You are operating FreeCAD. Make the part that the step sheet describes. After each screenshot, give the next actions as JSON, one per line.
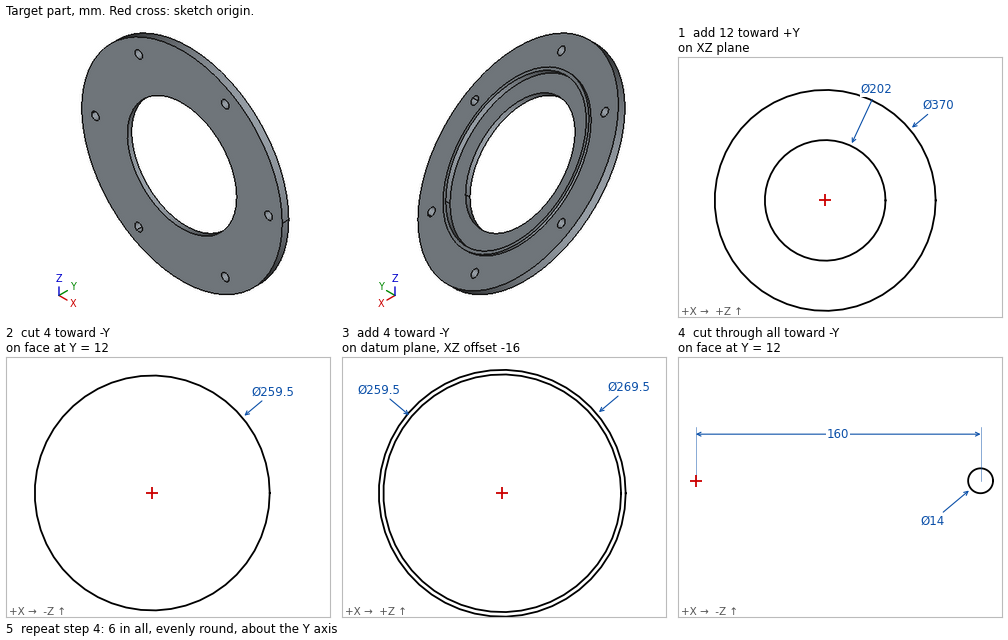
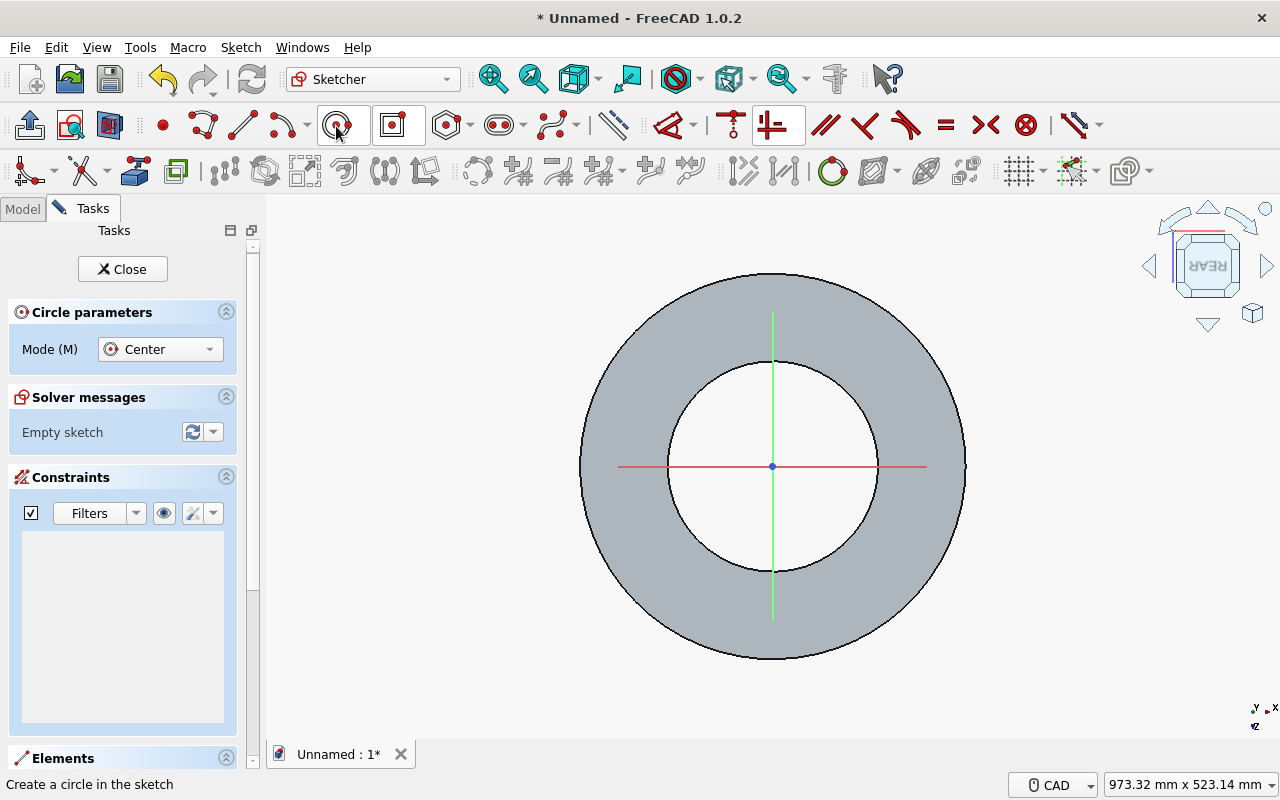
{"action": "left_click", "coordinate": [773, 466]}
{"action": "mouse_move", "coordinate": [868, 371]}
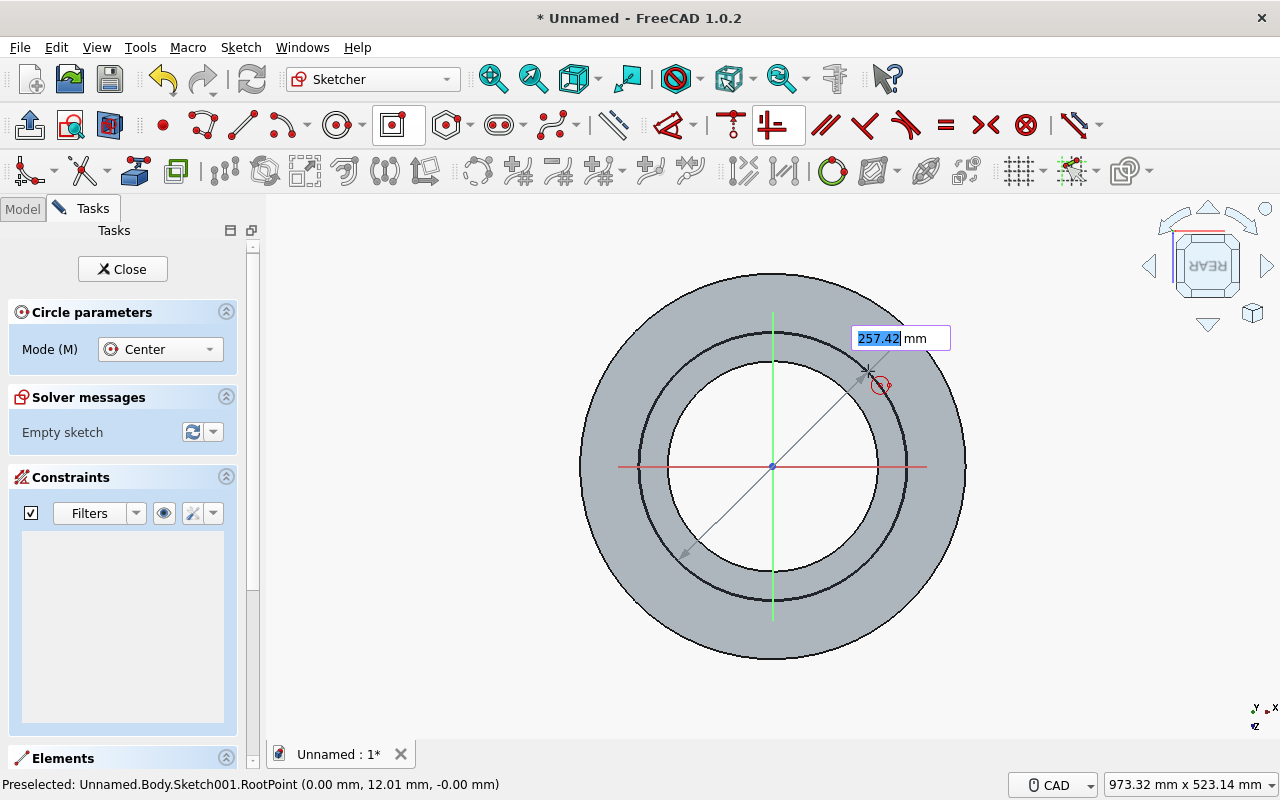
{"action": "type", "text": "259.5"}
{"action": "key", "text": "Return"}
{"action": "key", "text": "Escape"}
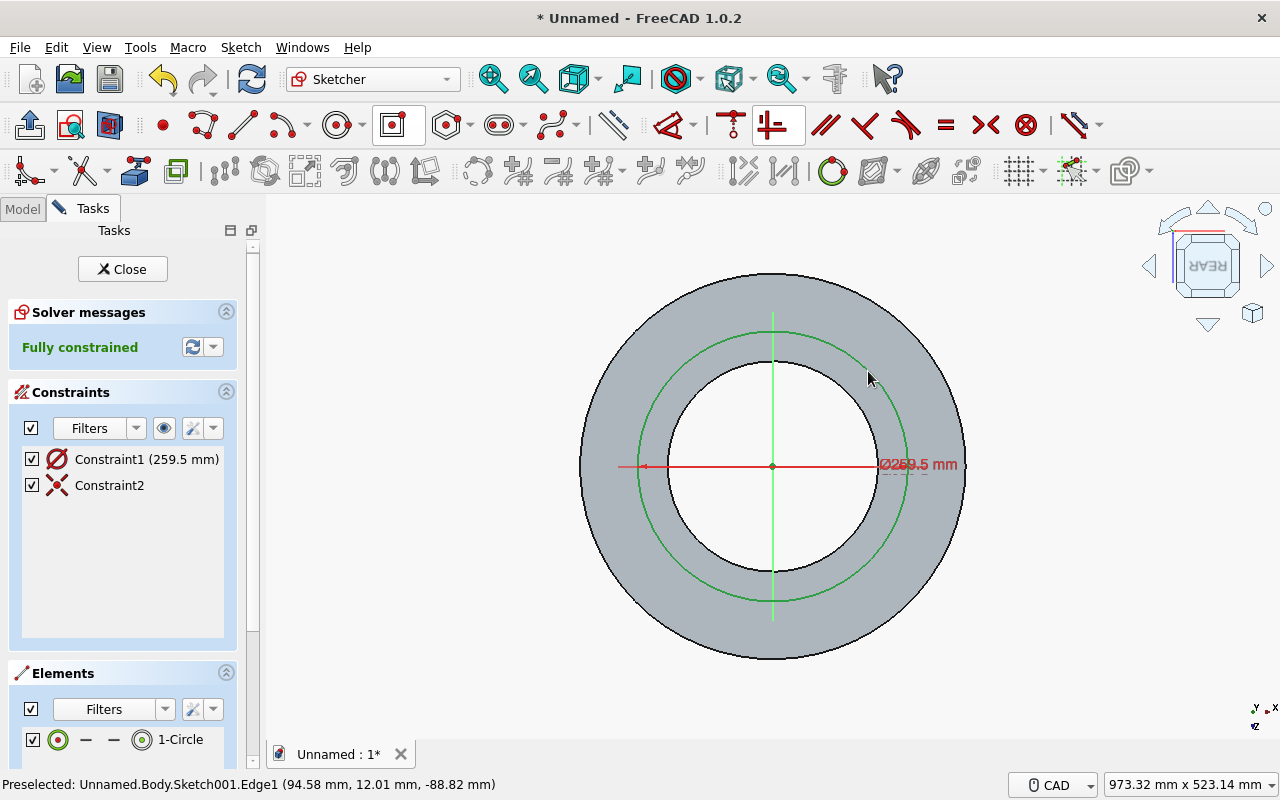
{"action": "left_click", "coordinate": [123, 269]}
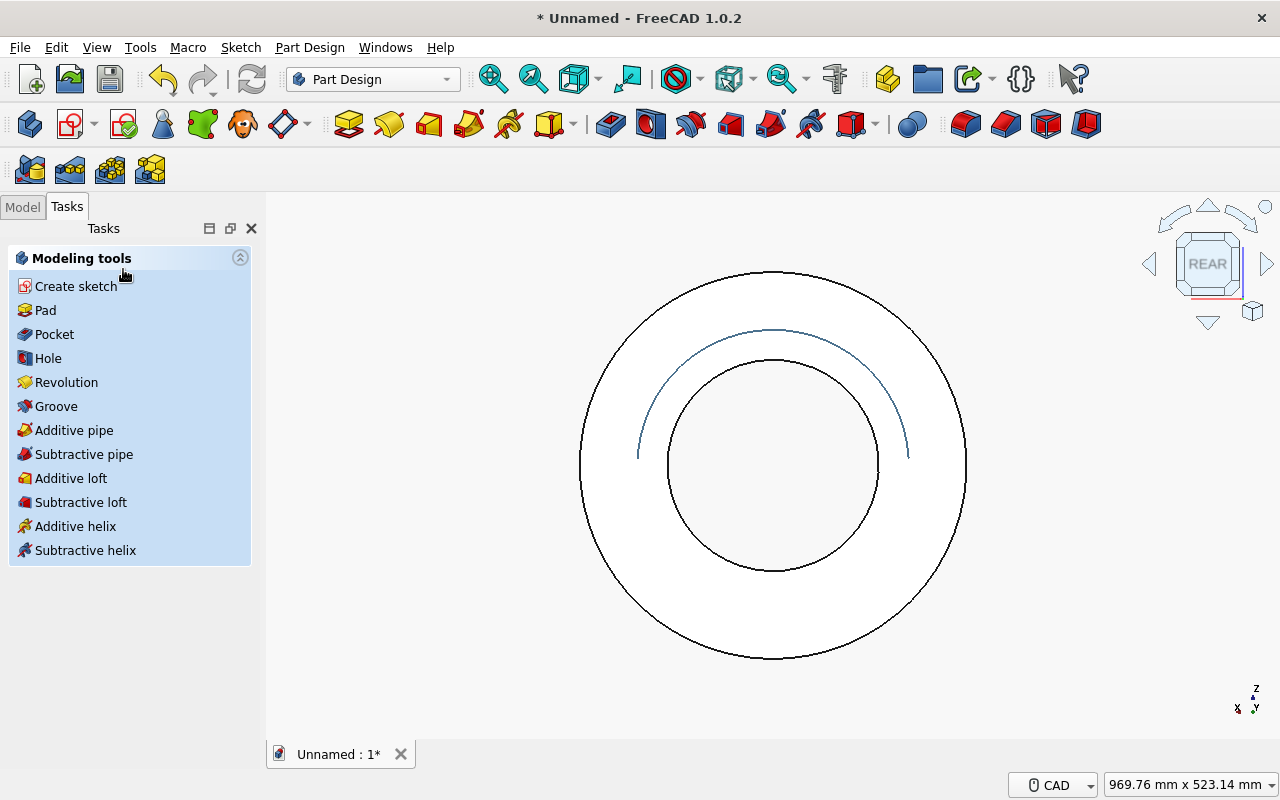
{"action": "left_click", "coordinate": [612, 124]}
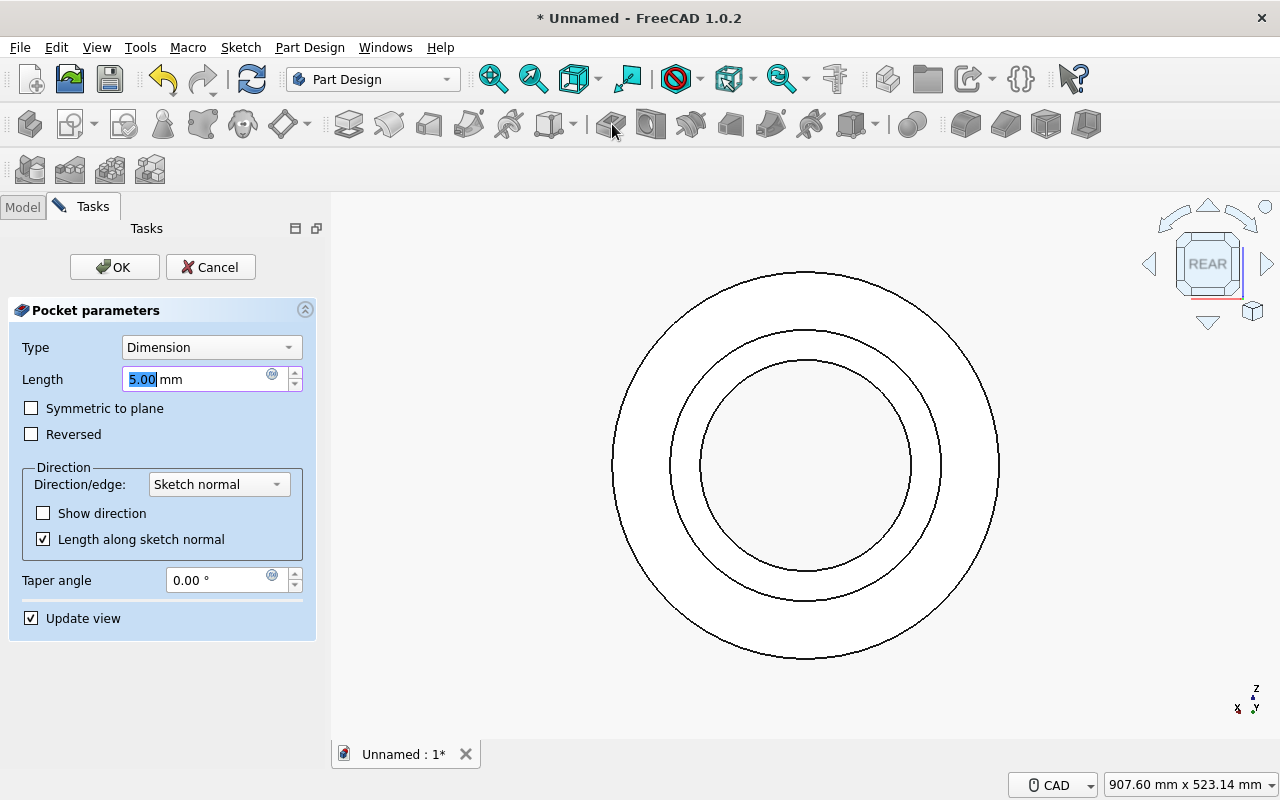
{"action": "type", "text": "4"}
{"action": "key", "text": "Tab"}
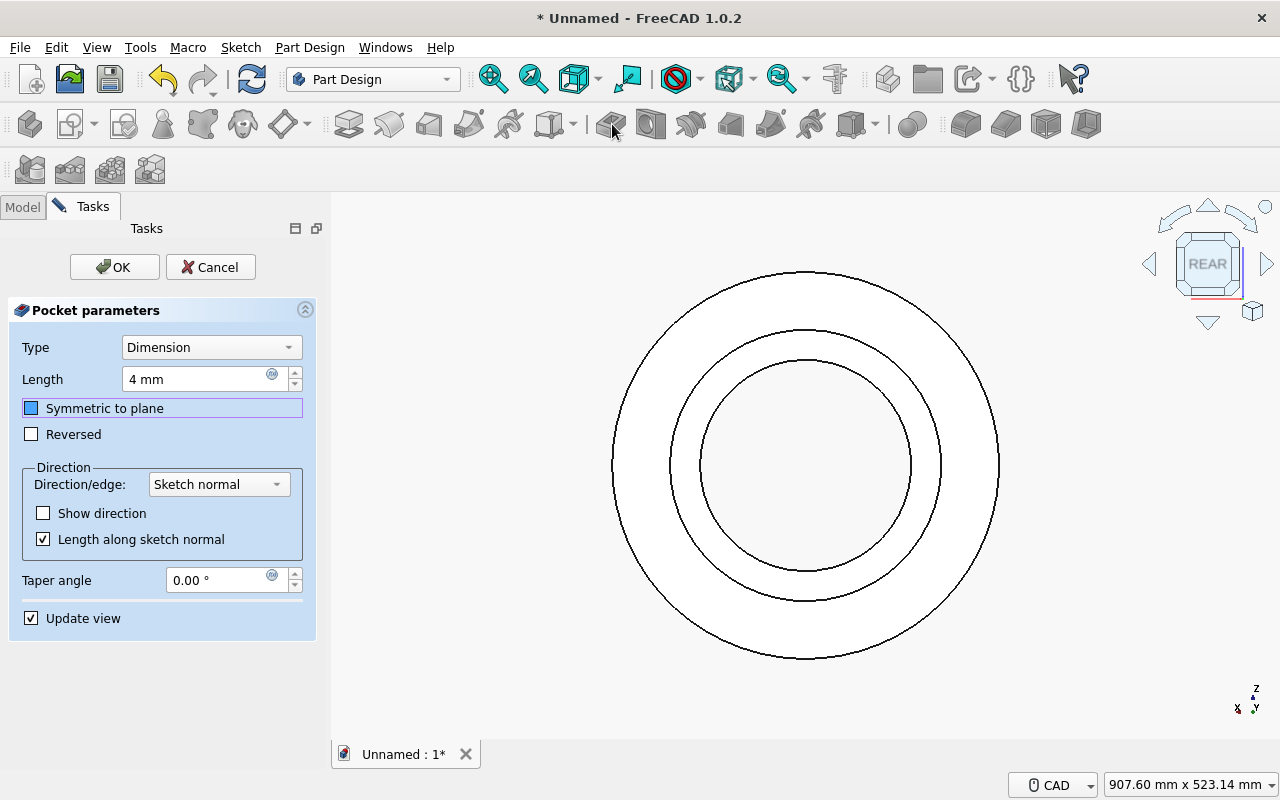
{"action": "left_click", "coordinate": [115, 267]}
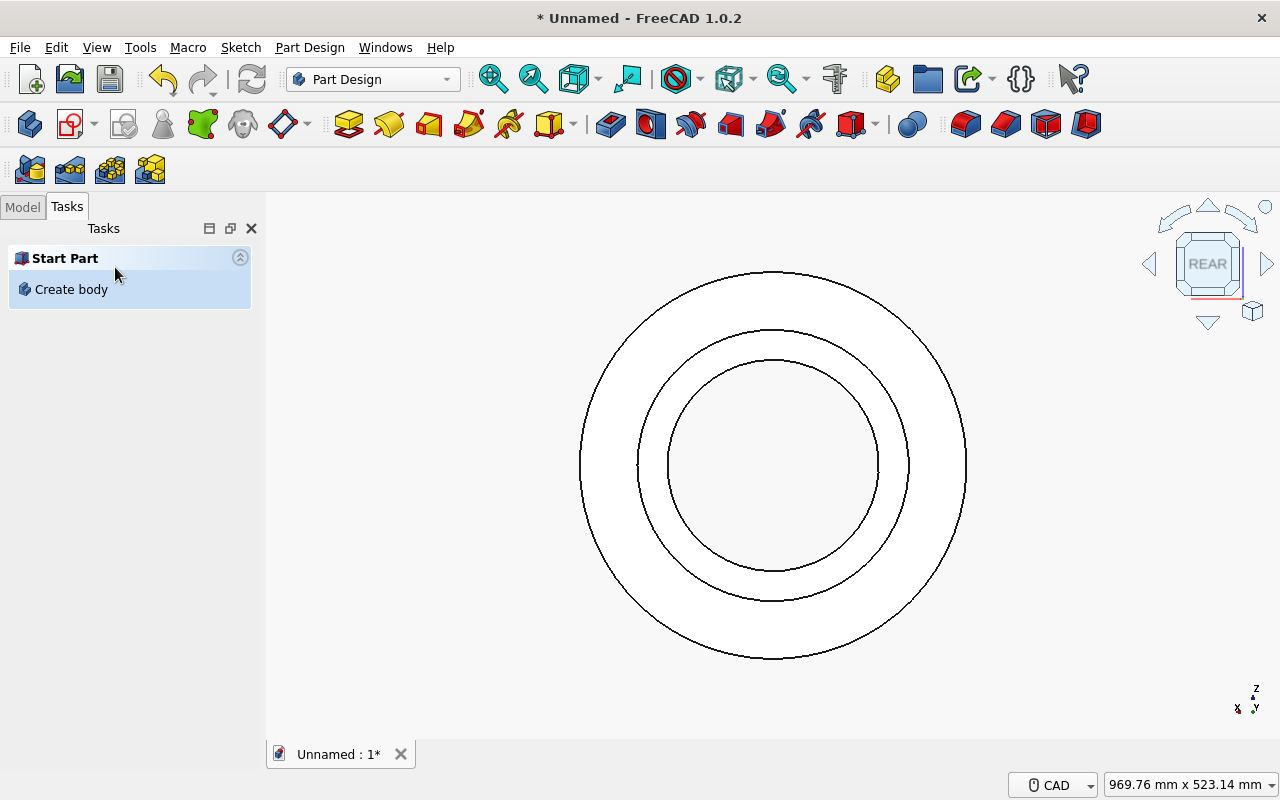
{"action": "left_click", "coordinate": [23, 206]}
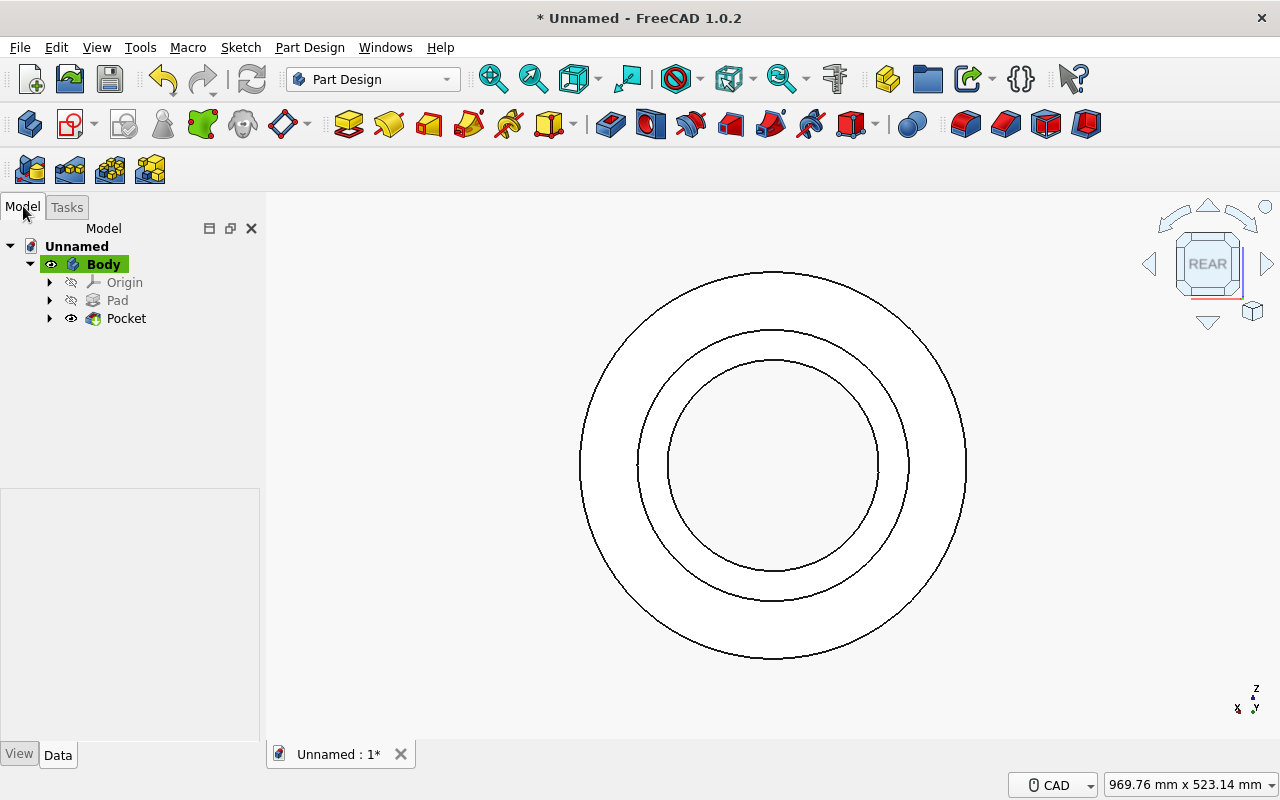
{"action": "left_click", "coordinate": [50, 282]}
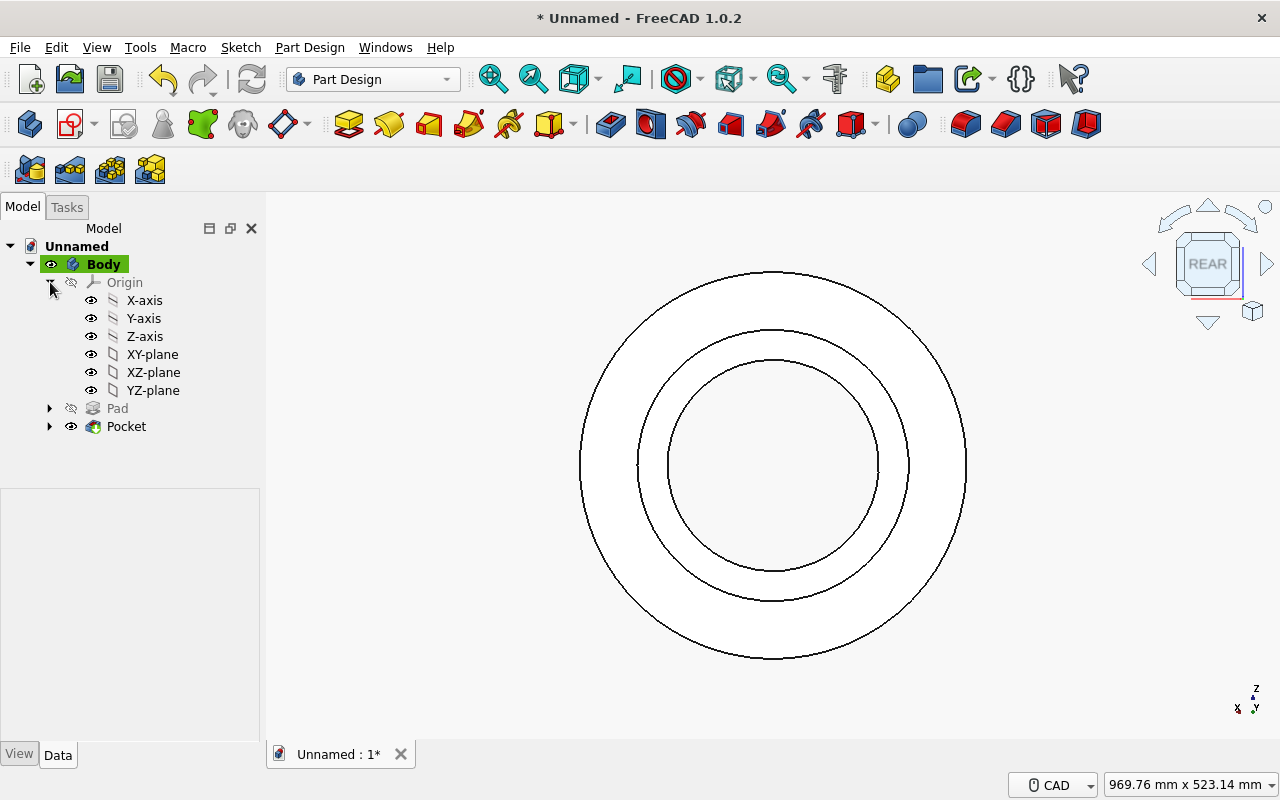
{"action": "left_click", "coordinate": [136, 372]}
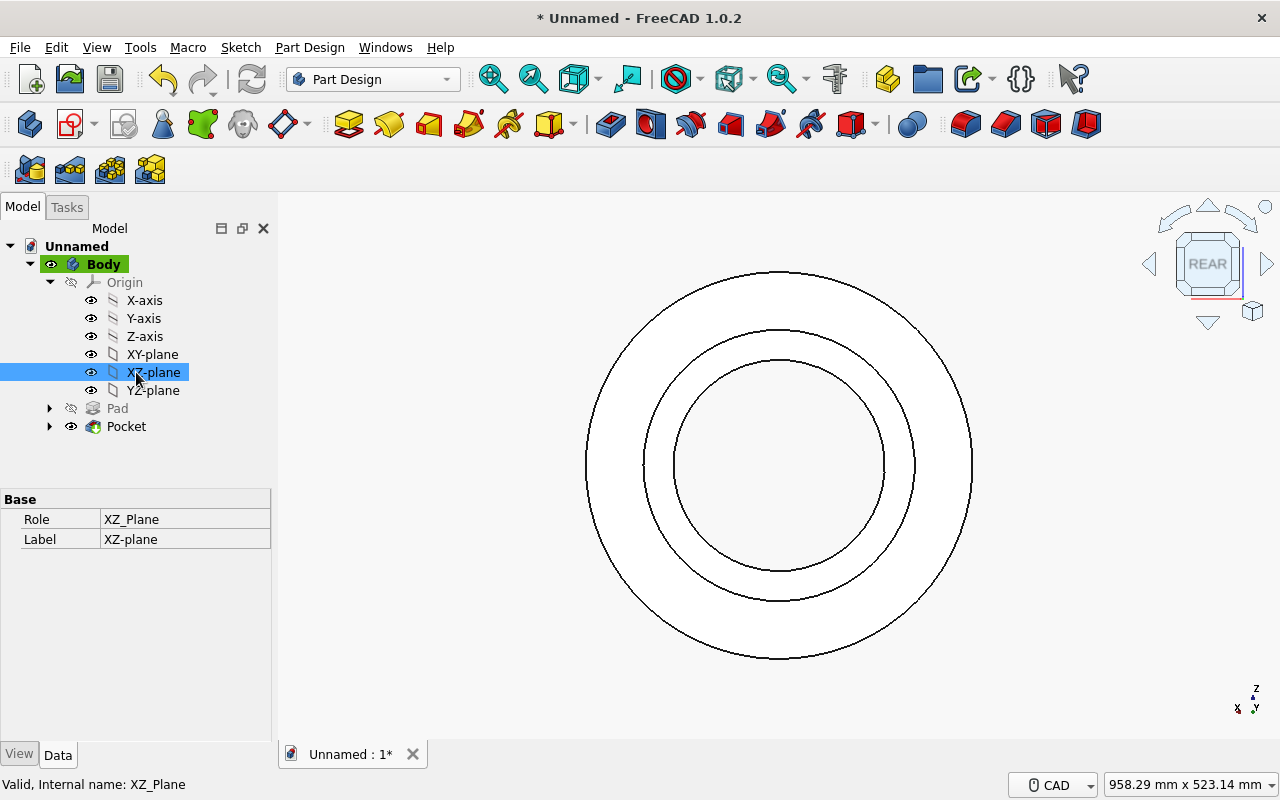
{"action": "left_click", "coordinate": [284, 124]}